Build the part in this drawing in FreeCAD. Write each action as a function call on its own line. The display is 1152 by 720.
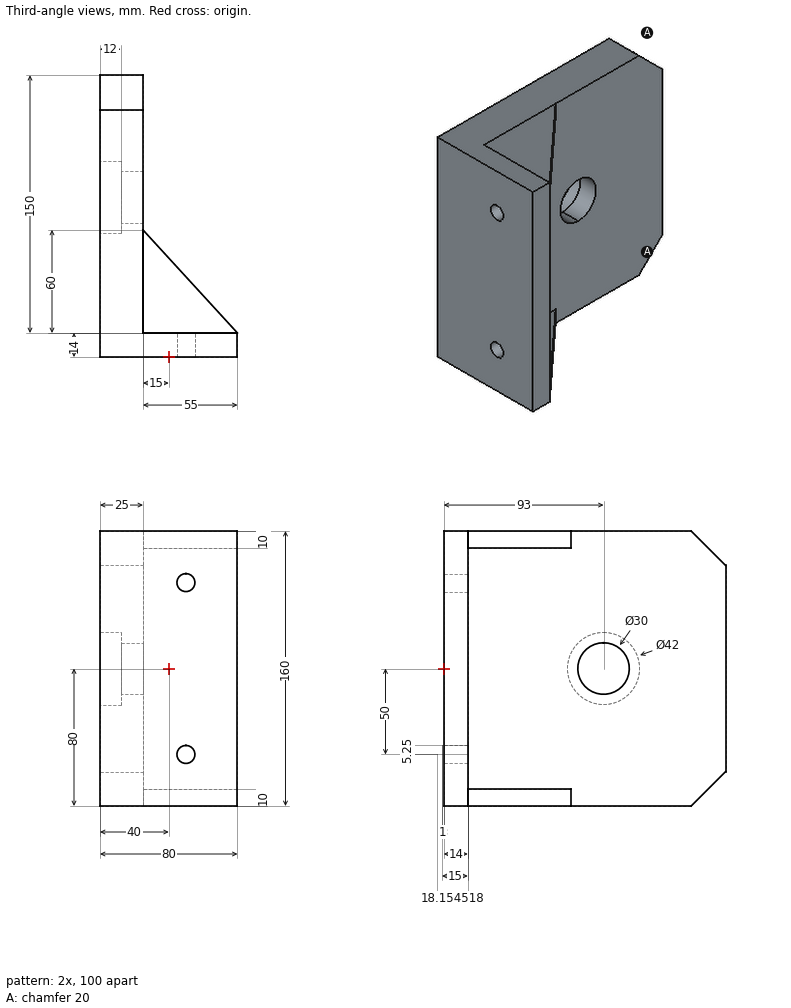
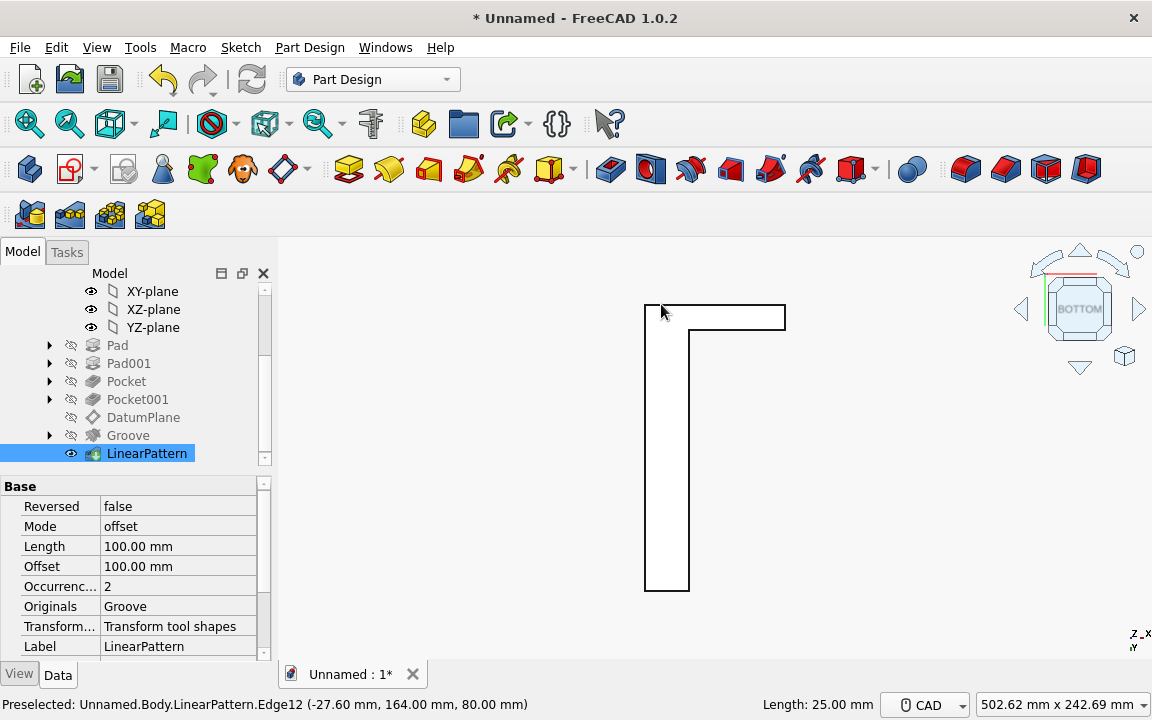
key(4)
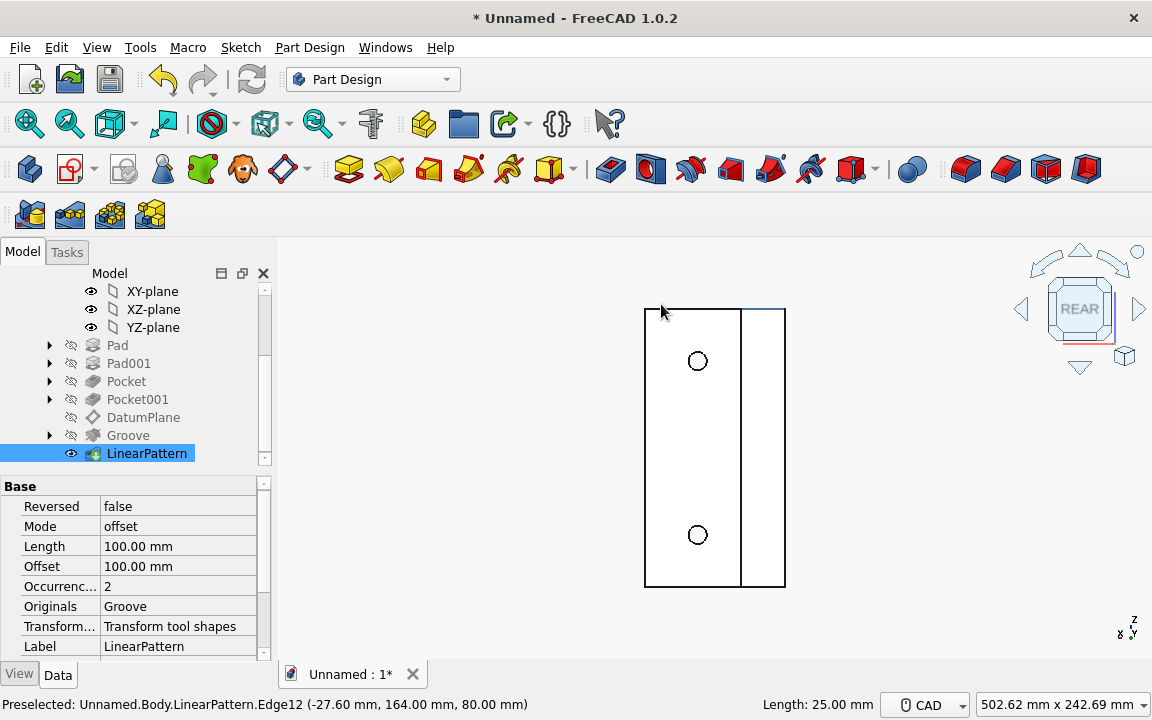
click(763, 586, ctrl)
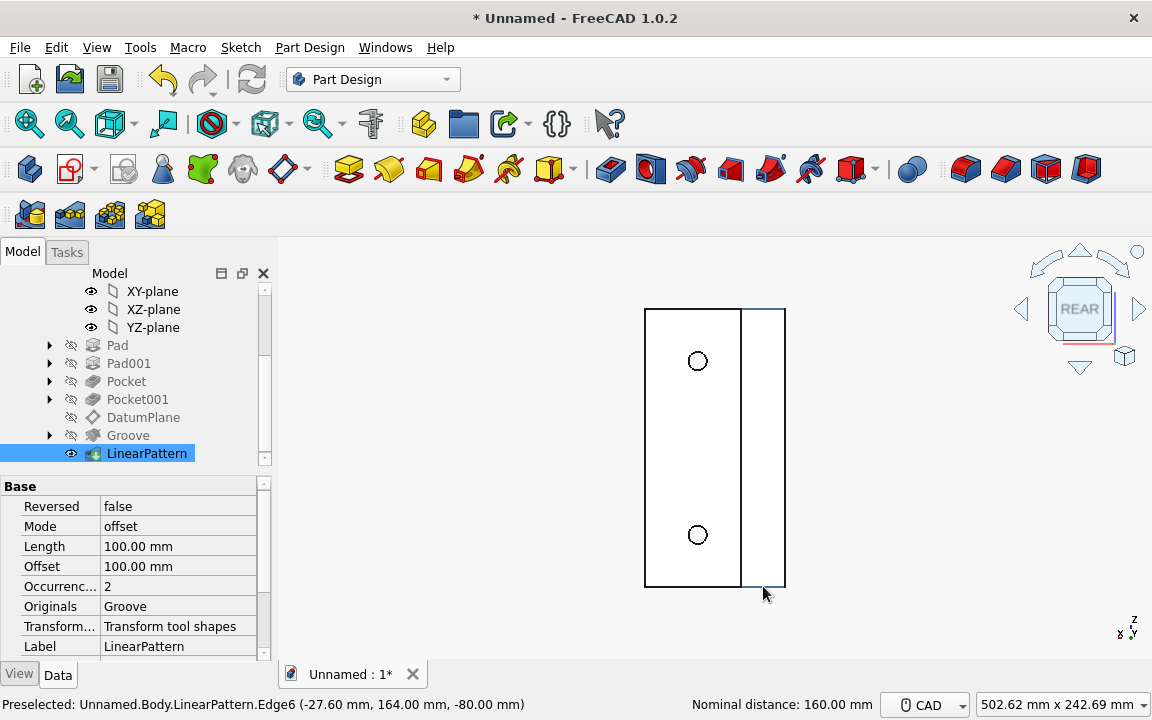
click(1006, 170)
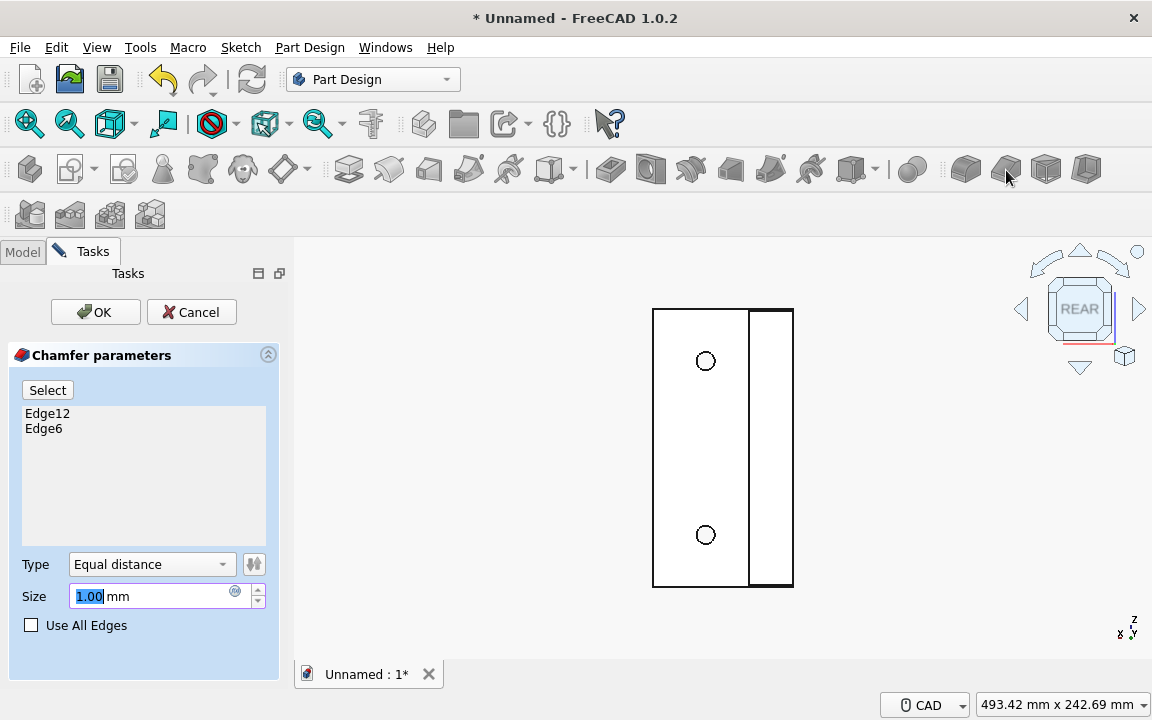
text(20)
key(Tab)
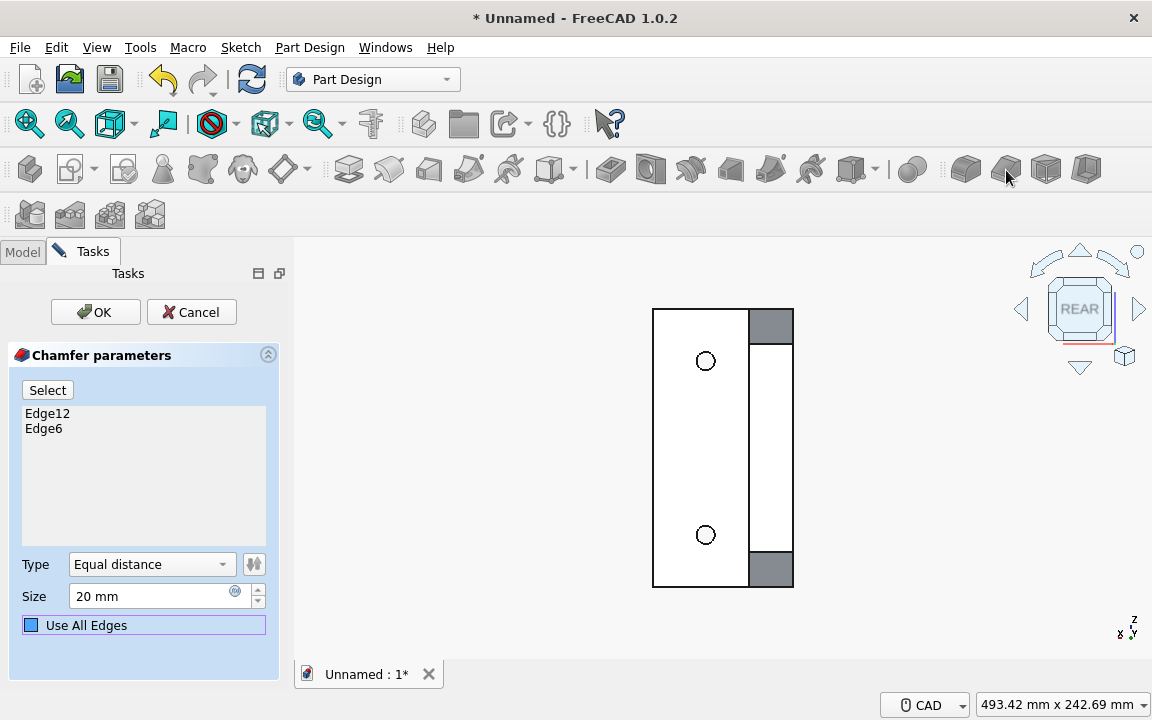
click(96, 312)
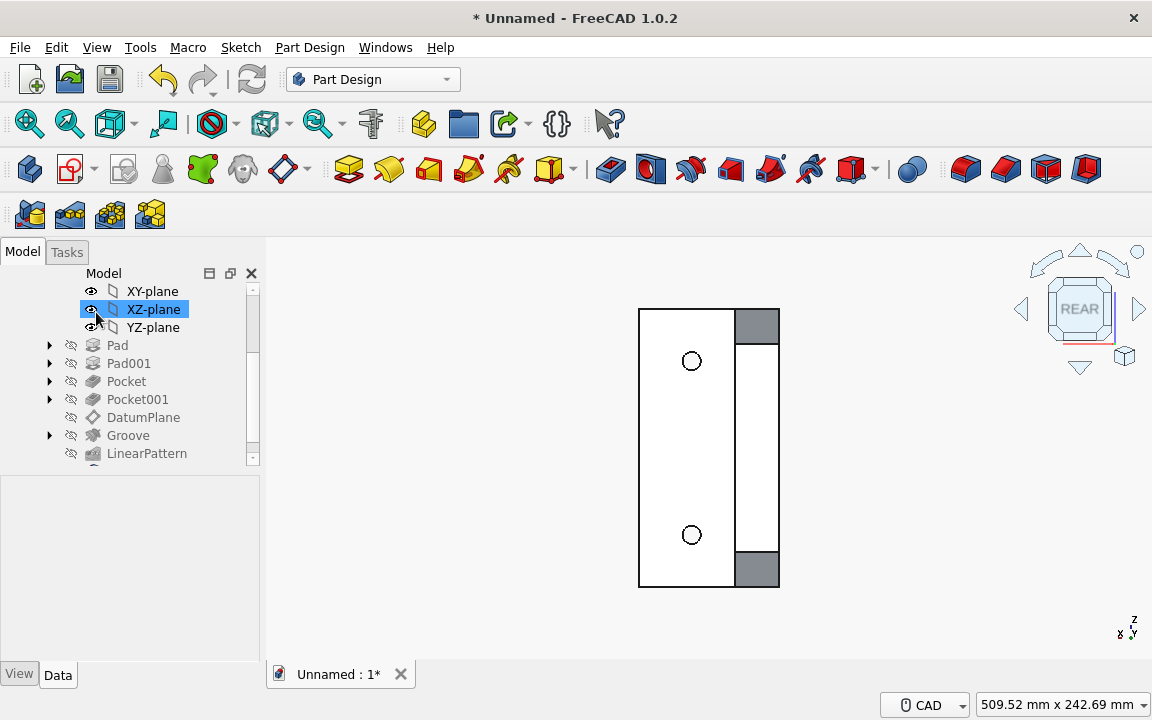
click(30, 170)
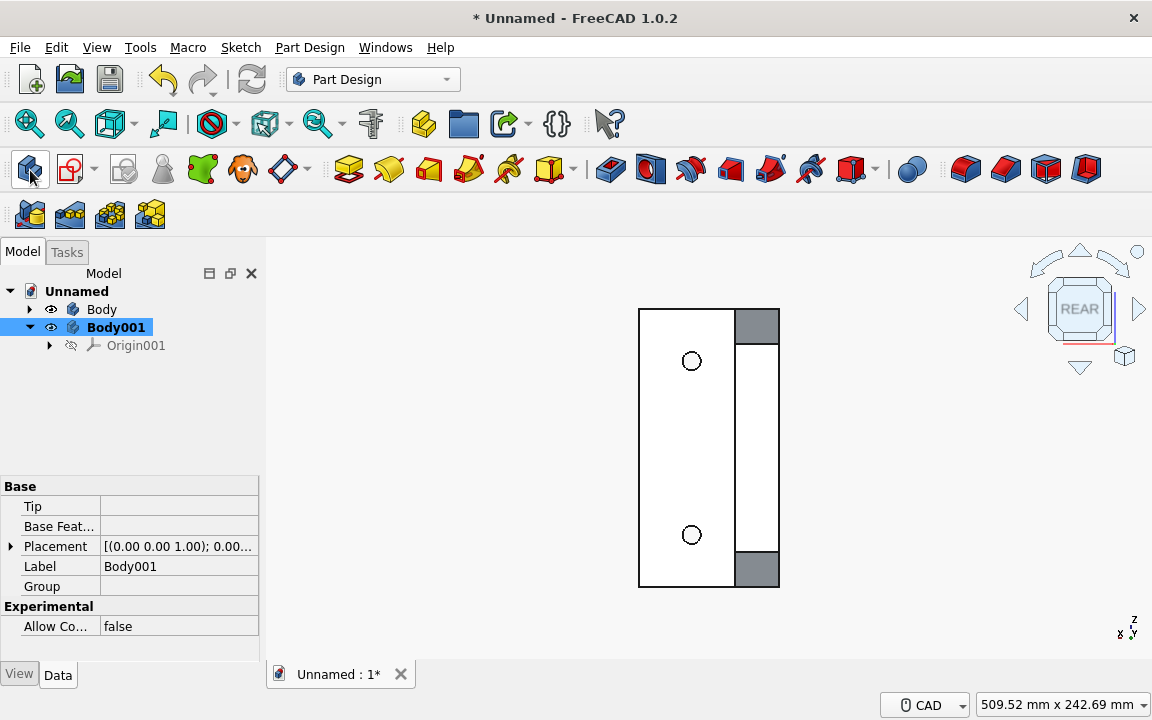
click(50, 345)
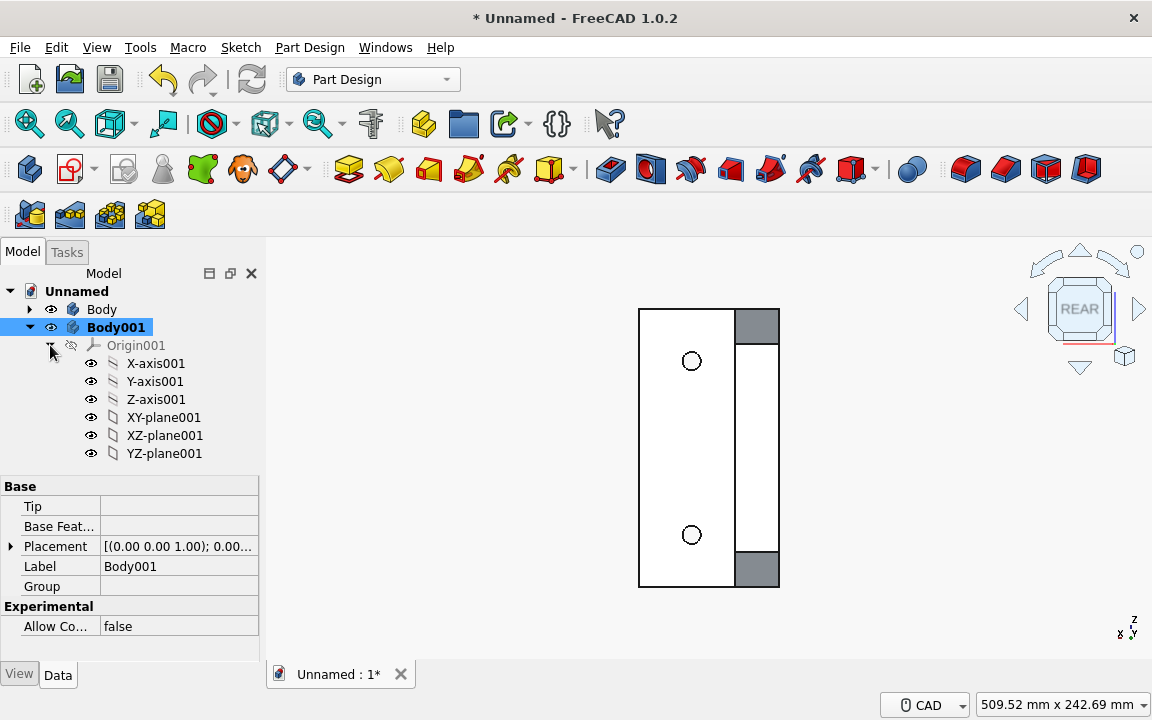
click(136, 417)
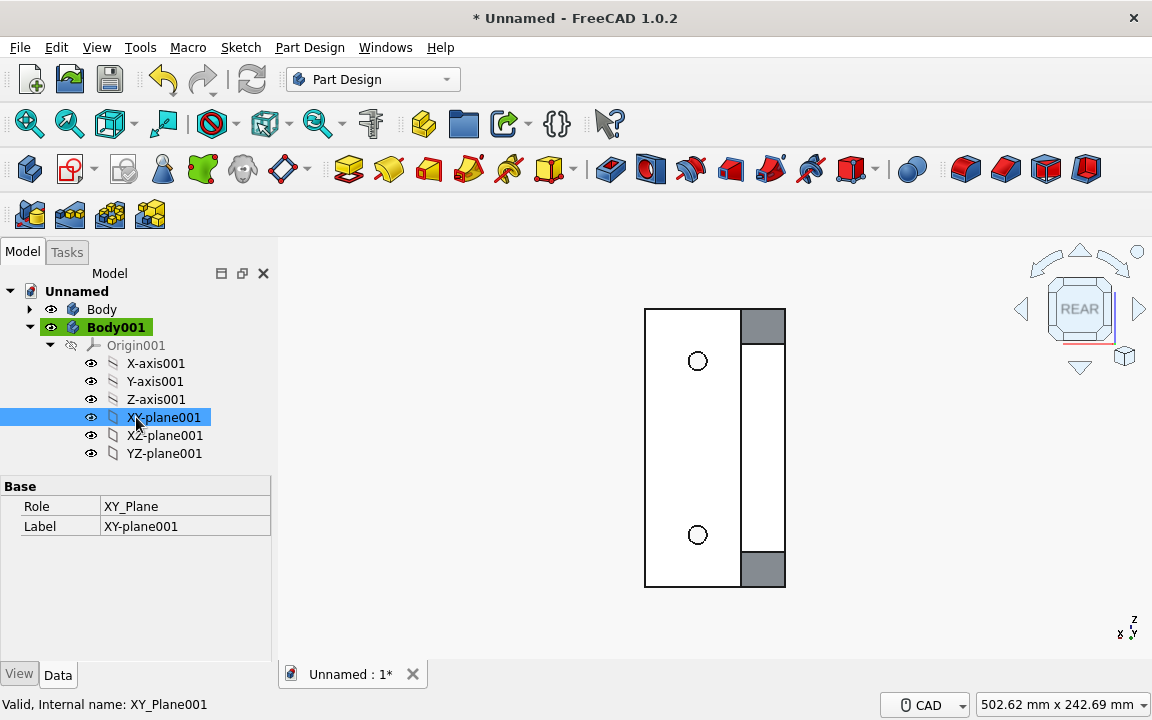
click(284, 170)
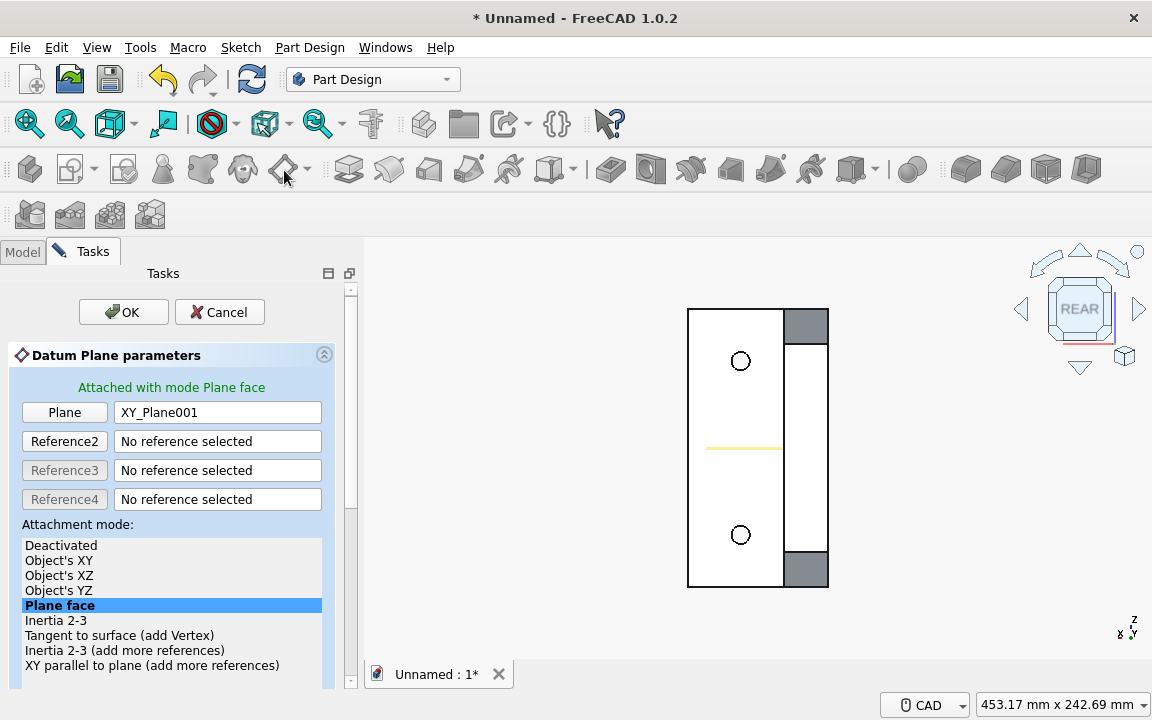
scroll(351, 486, down, 4)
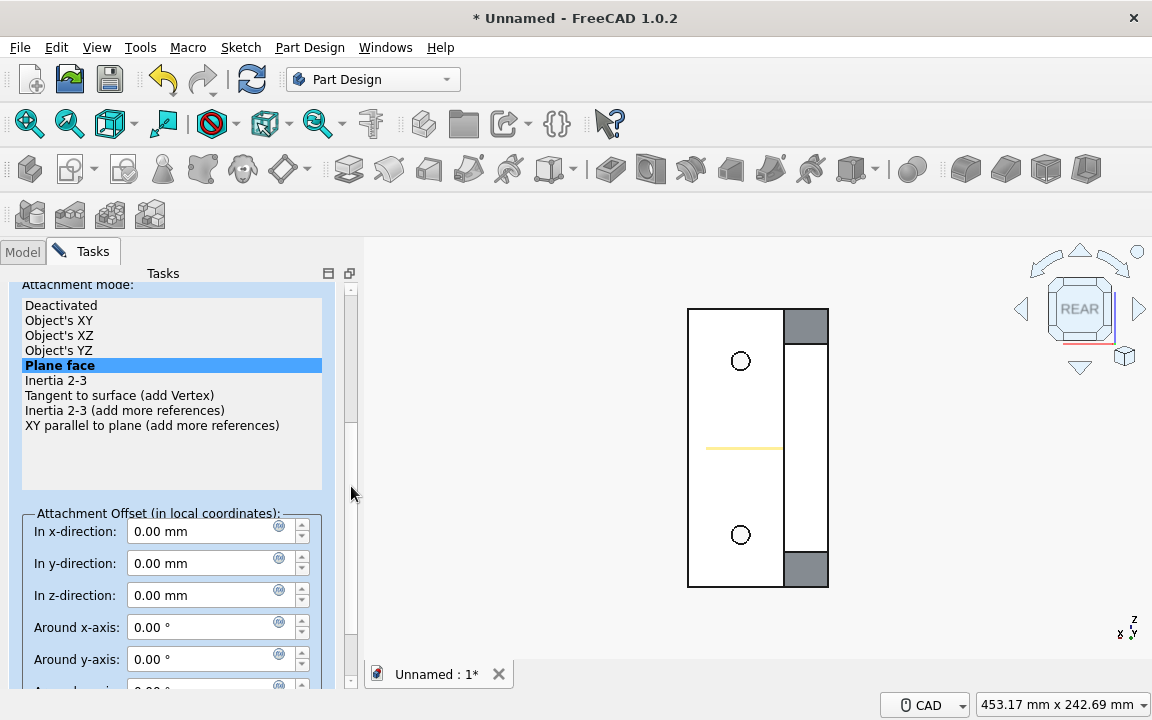
triple_click(210, 595)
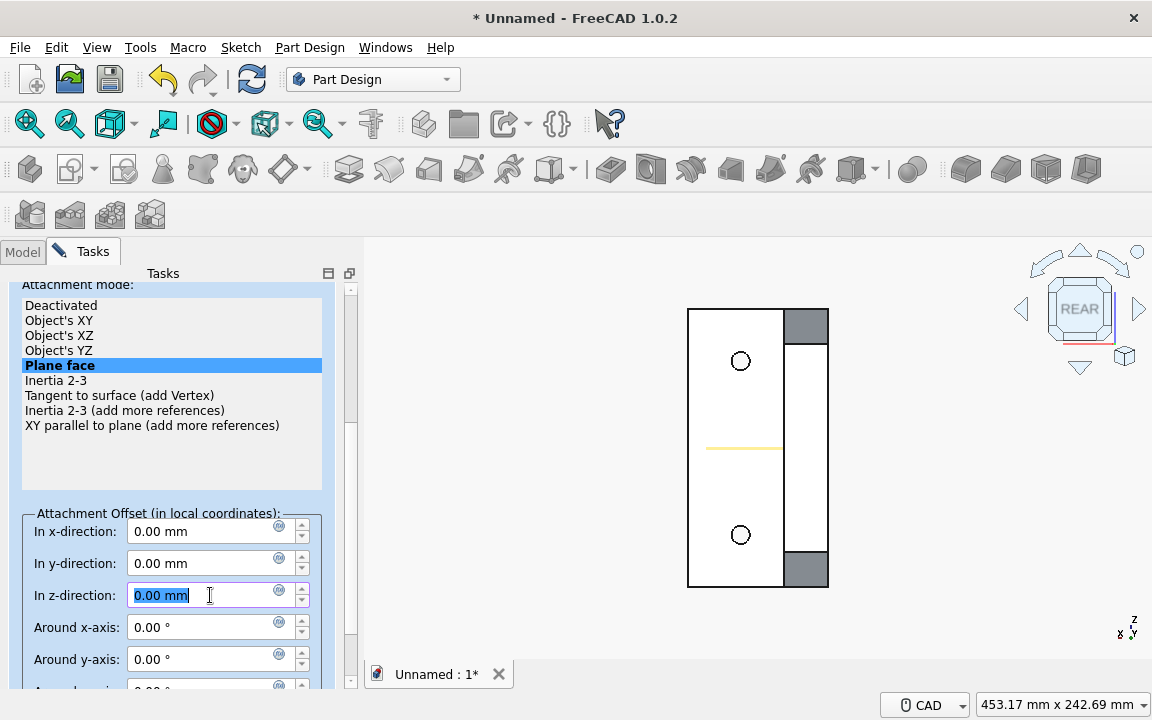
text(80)
key(Tab)